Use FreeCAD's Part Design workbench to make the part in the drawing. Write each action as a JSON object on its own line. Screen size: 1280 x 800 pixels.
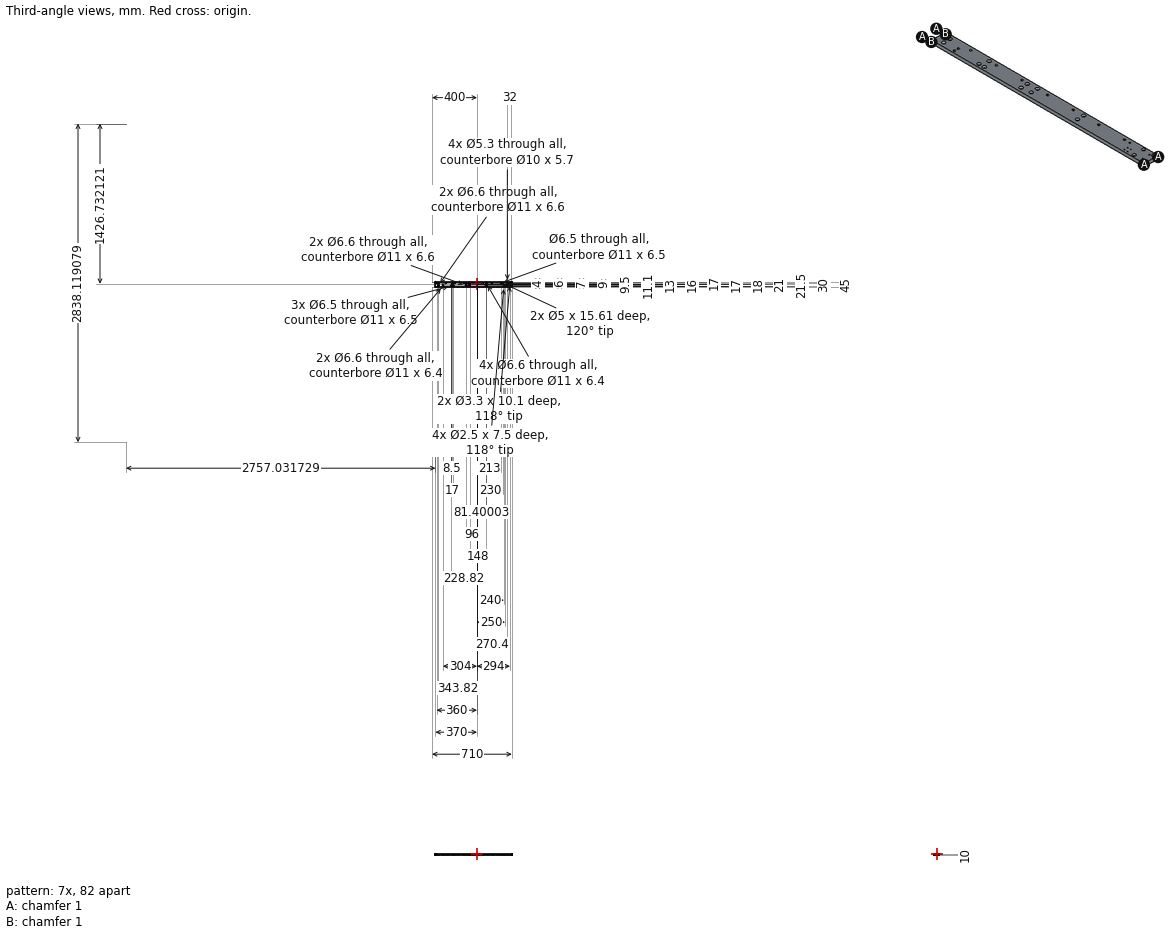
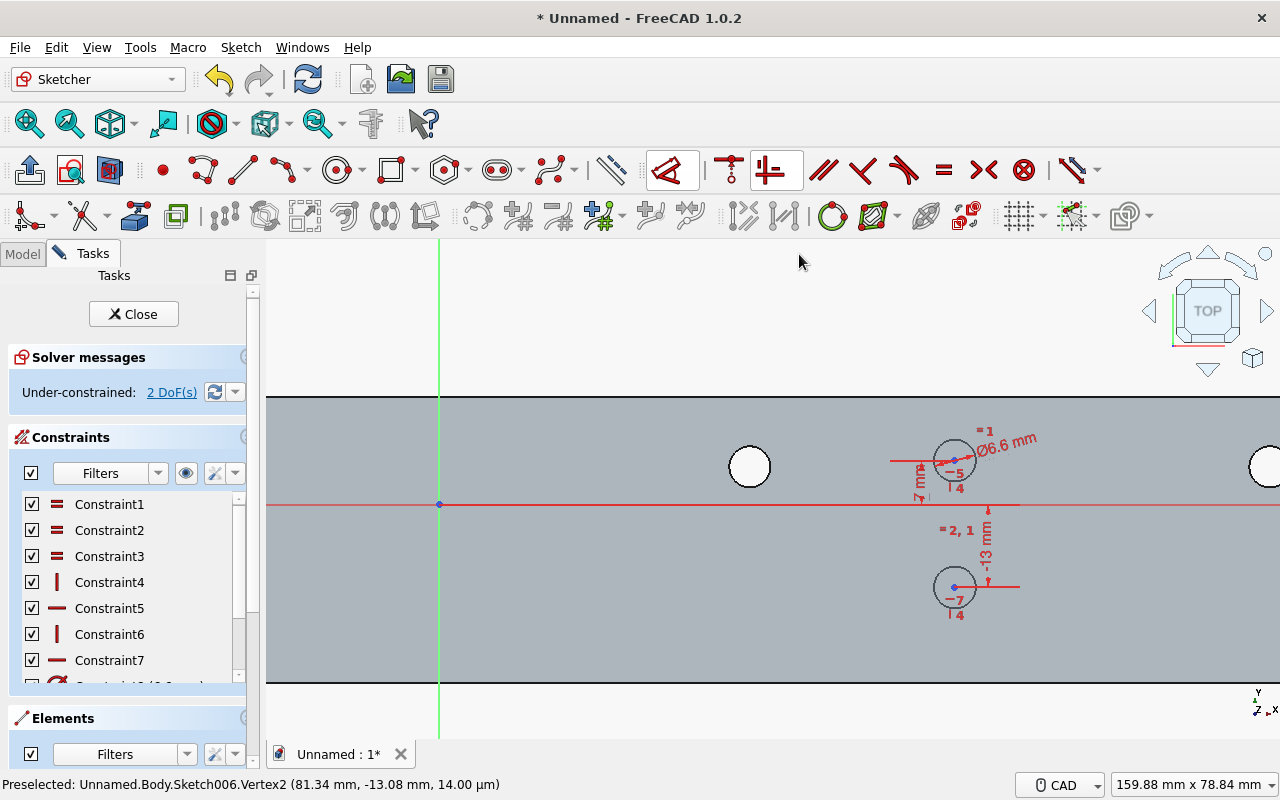
{"action": "left_click", "coordinate": [955, 461]}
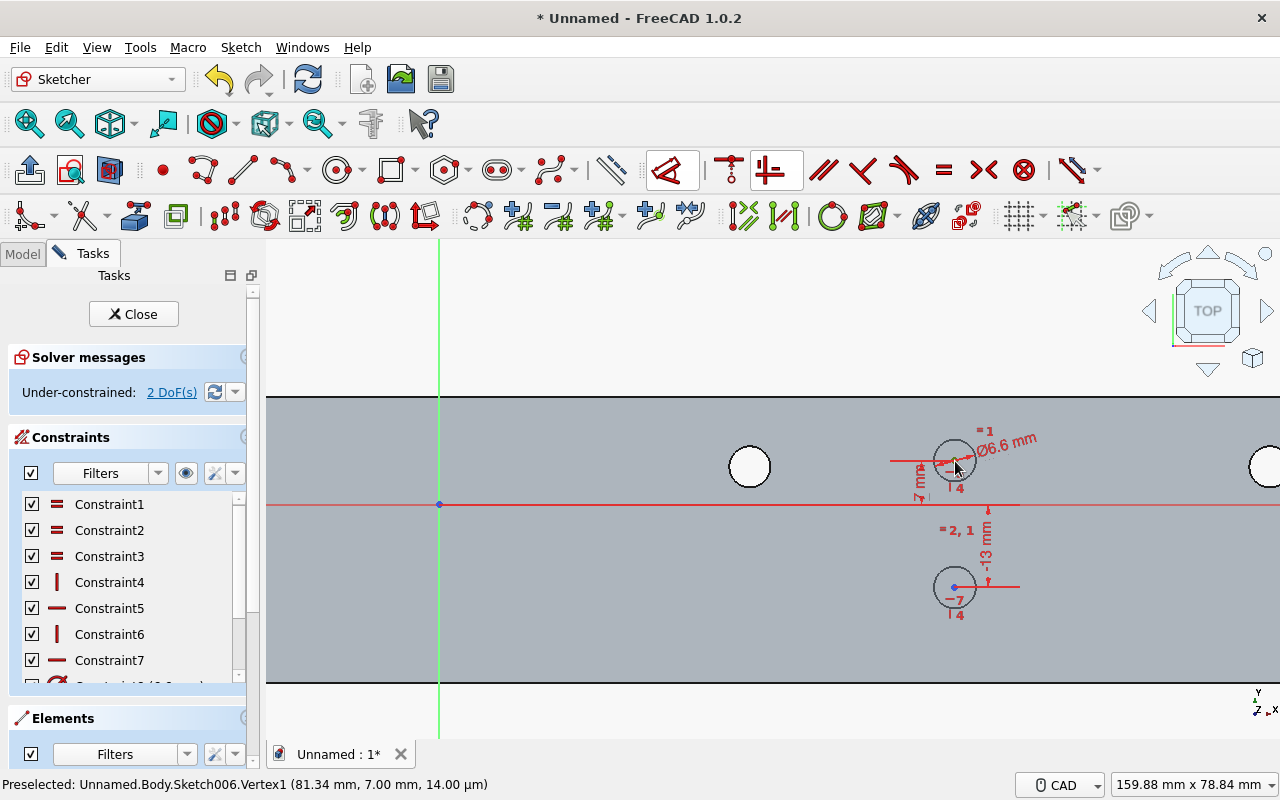
{"action": "scroll", "coordinate": [970, 446], "scroll_direction": "down", "scroll_amount": 3}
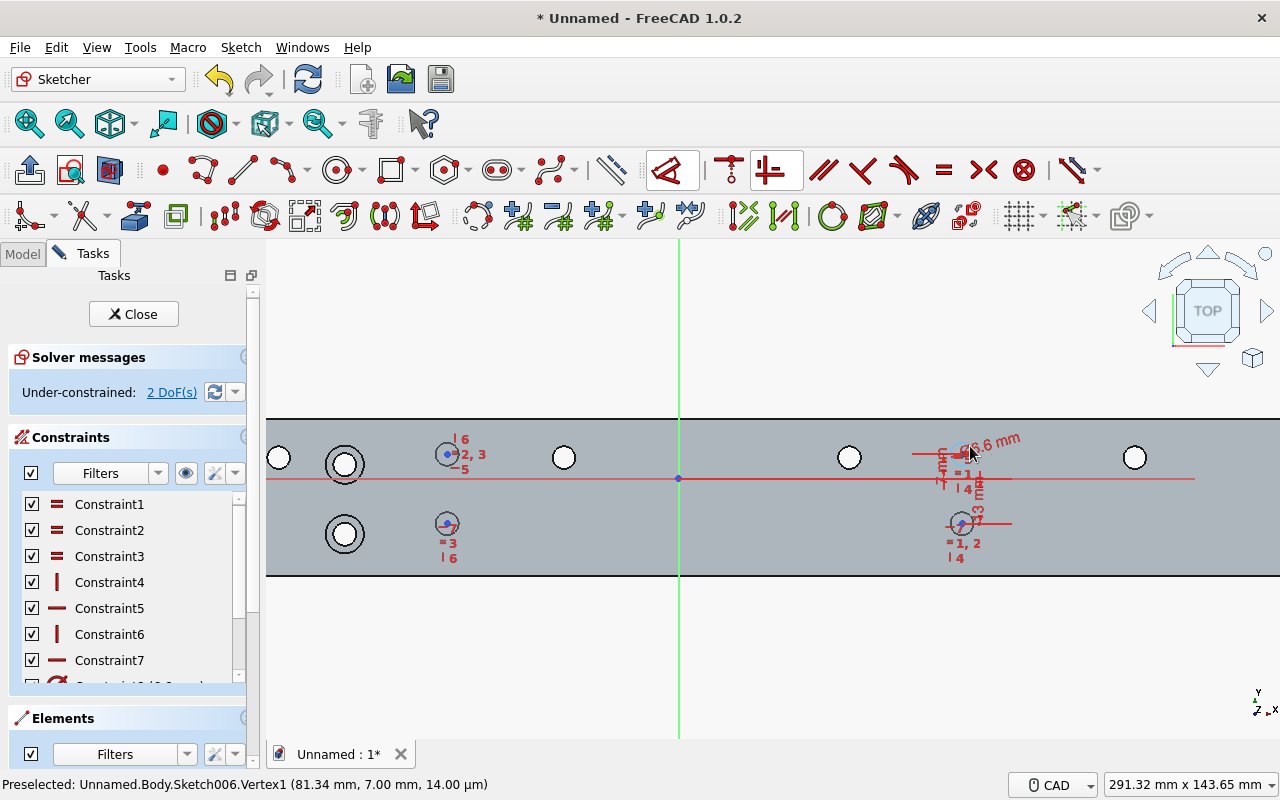
{"action": "left_click", "coordinate": [447, 454]}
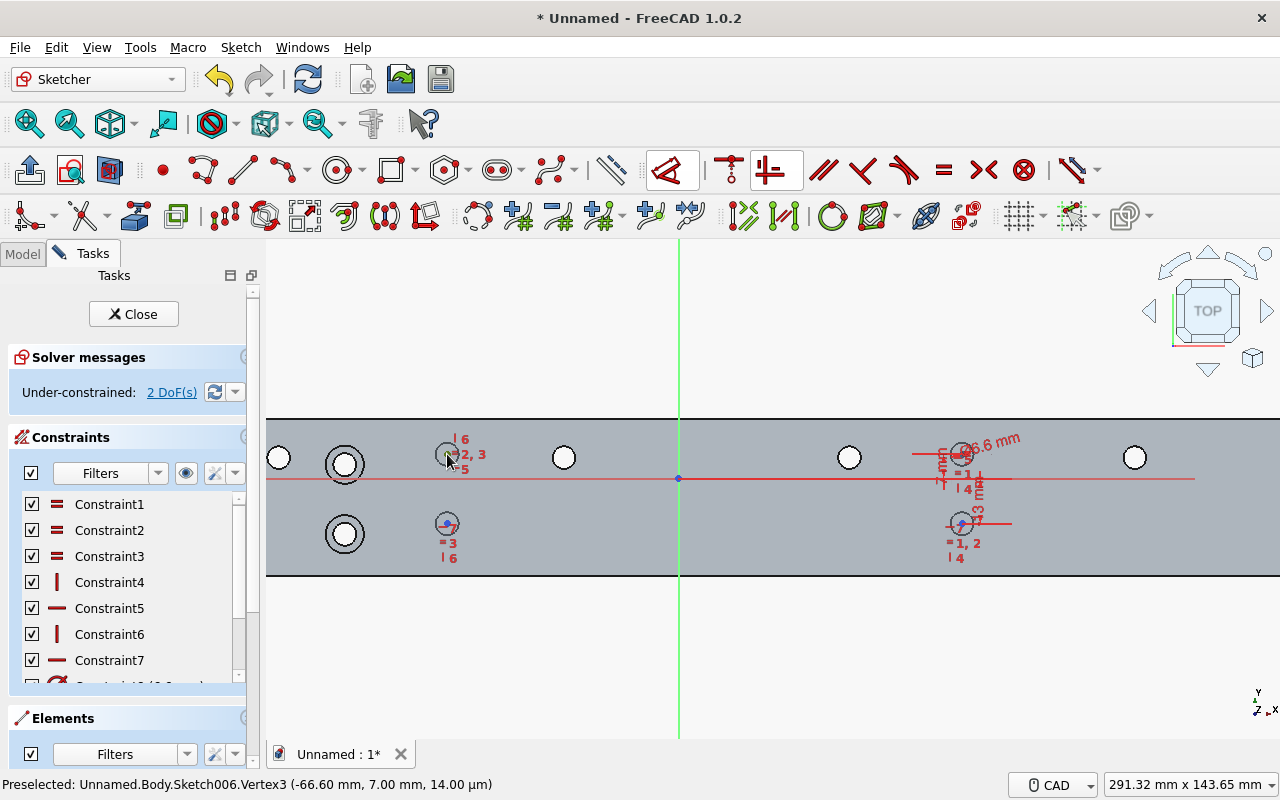
{"action": "left_click", "coordinate": [694, 170]}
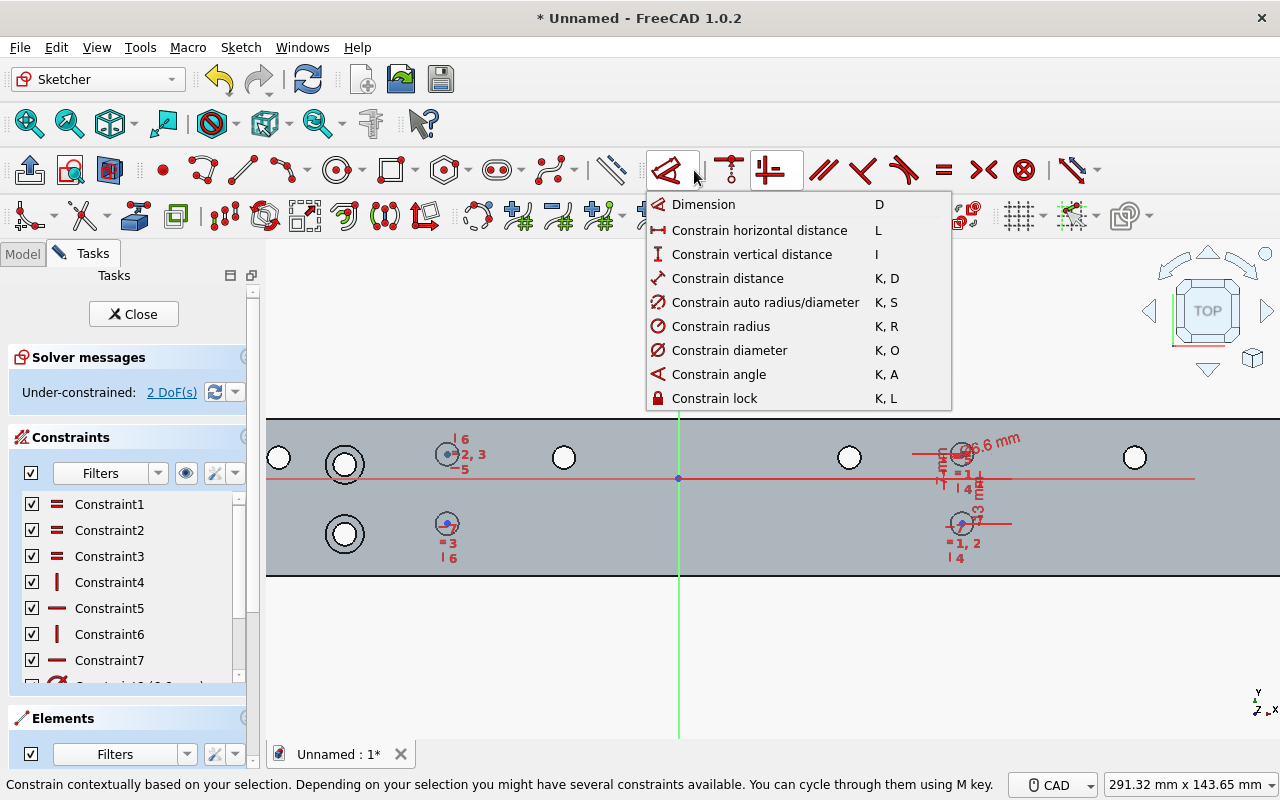
{"action": "left_click", "coordinate": [799, 230]}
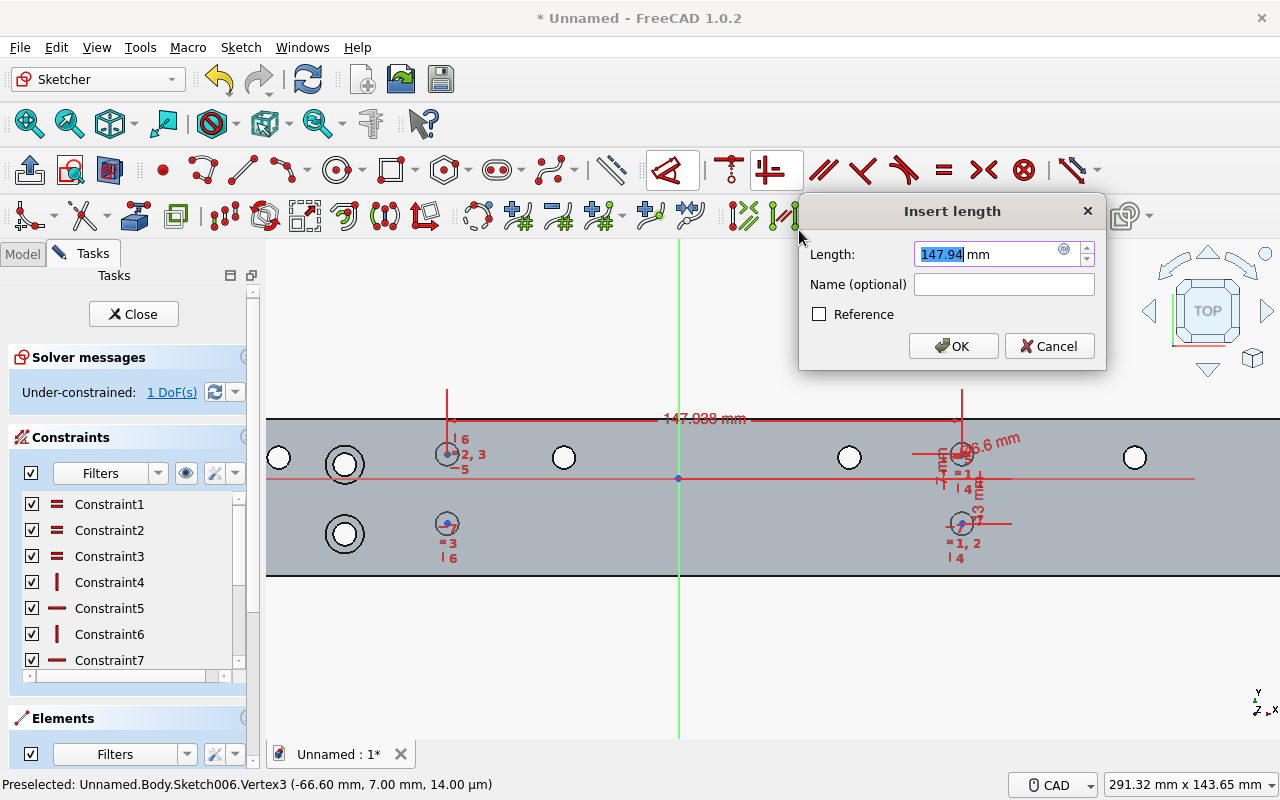
{"action": "type", "text": "148"}
{"action": "key", "text": "Return"}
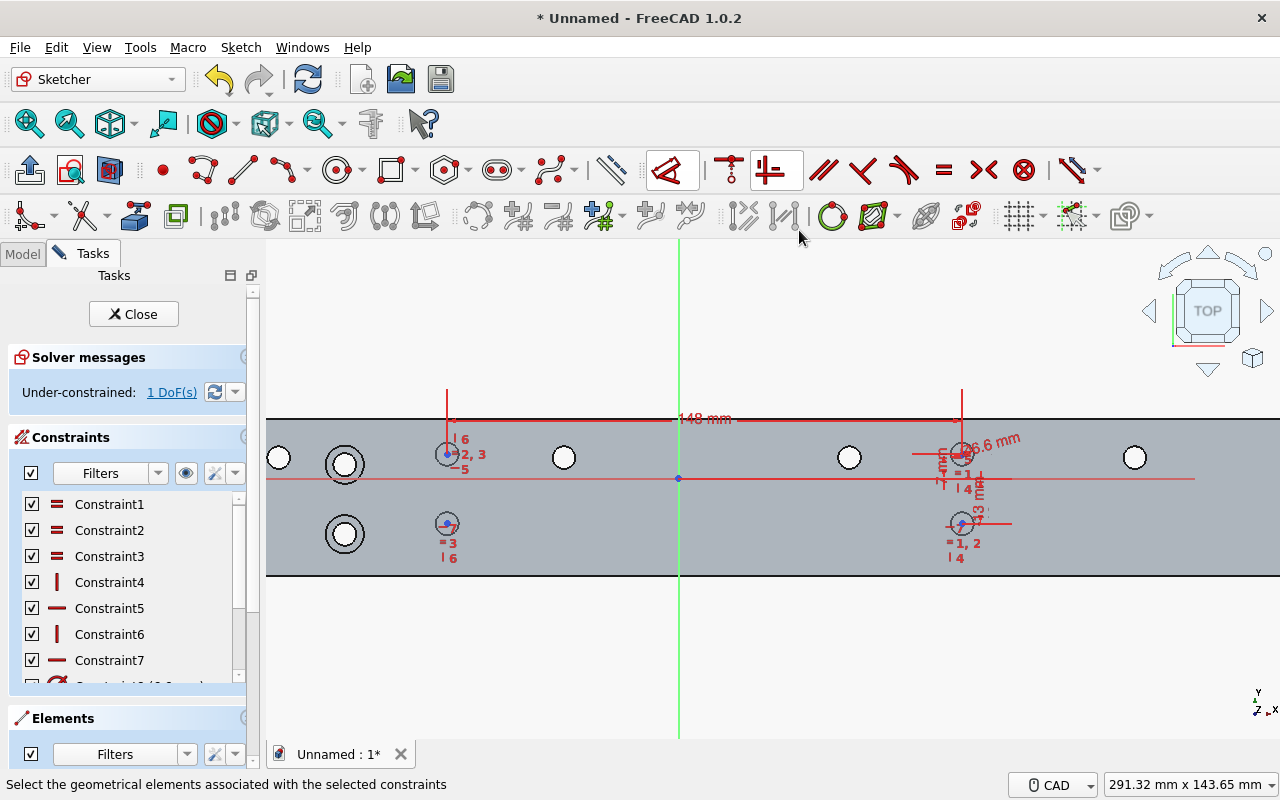
{"action": "left_click", "coordinate": [962, 454]}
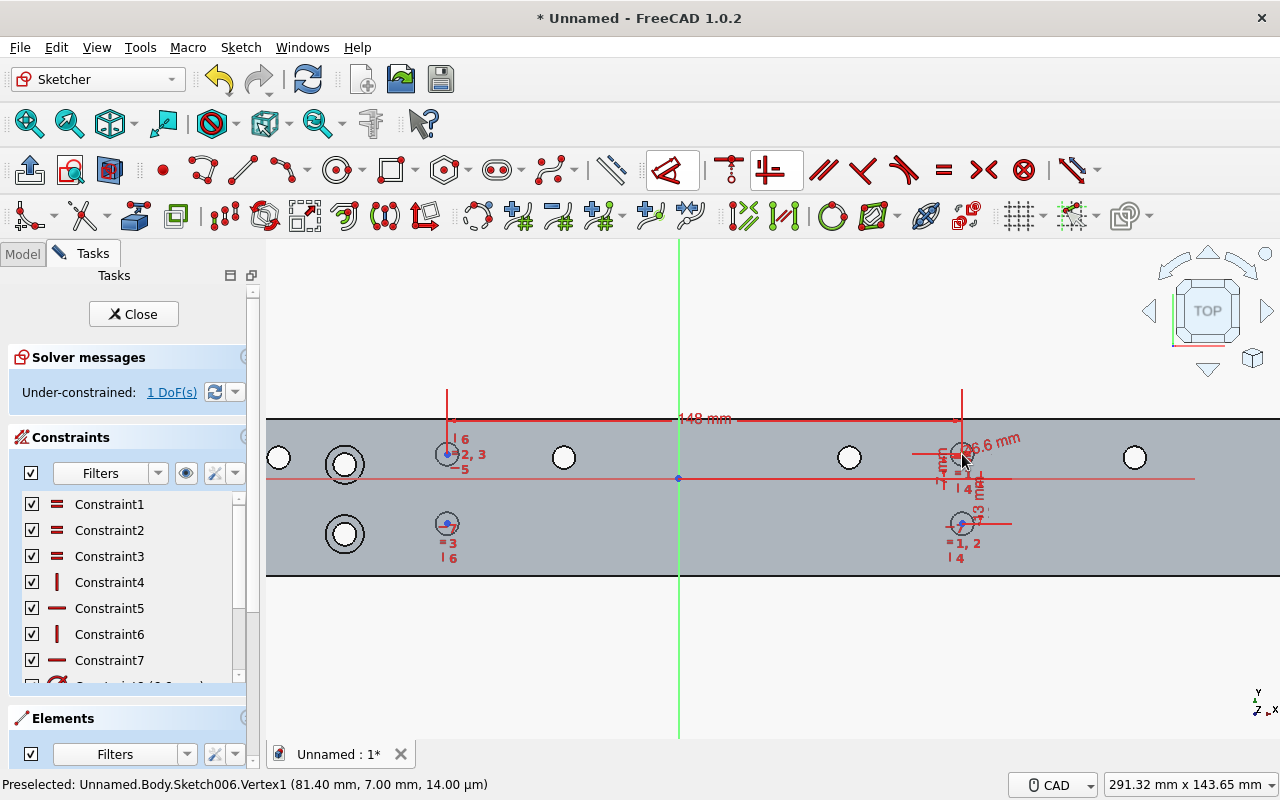
{"action": "left_click", "coordinate": [694, 170]}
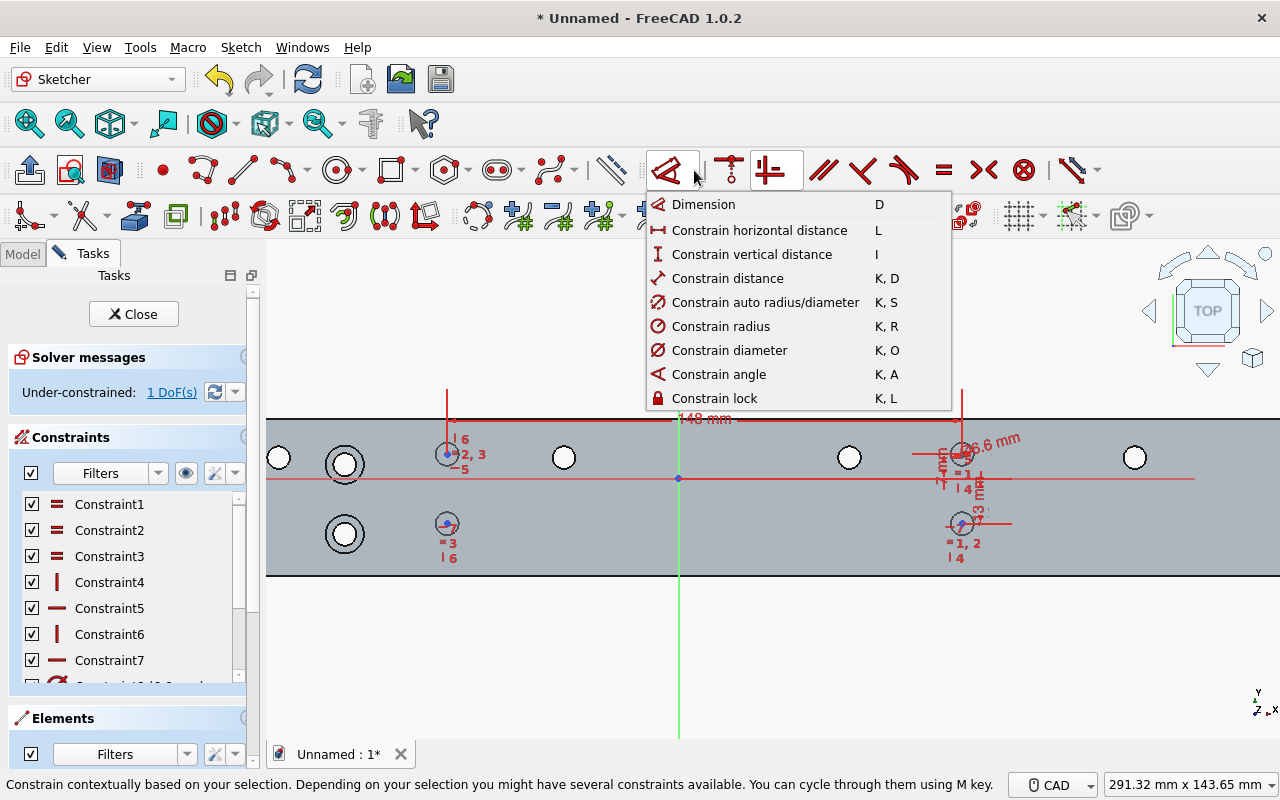
{"action": "left_click", "coordinate": [799, 230]}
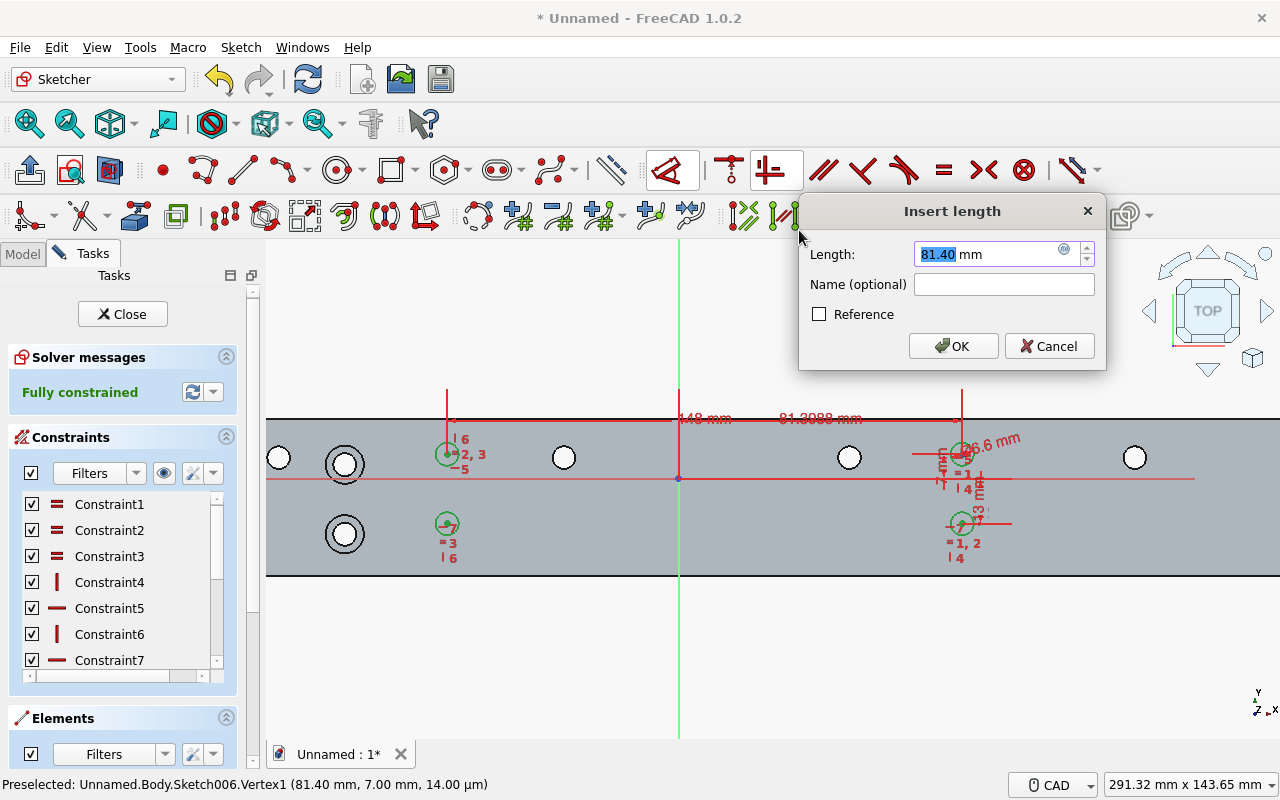
{"action": "type", "text": "81.40003"}
{"action": "key", "text": "Return"}